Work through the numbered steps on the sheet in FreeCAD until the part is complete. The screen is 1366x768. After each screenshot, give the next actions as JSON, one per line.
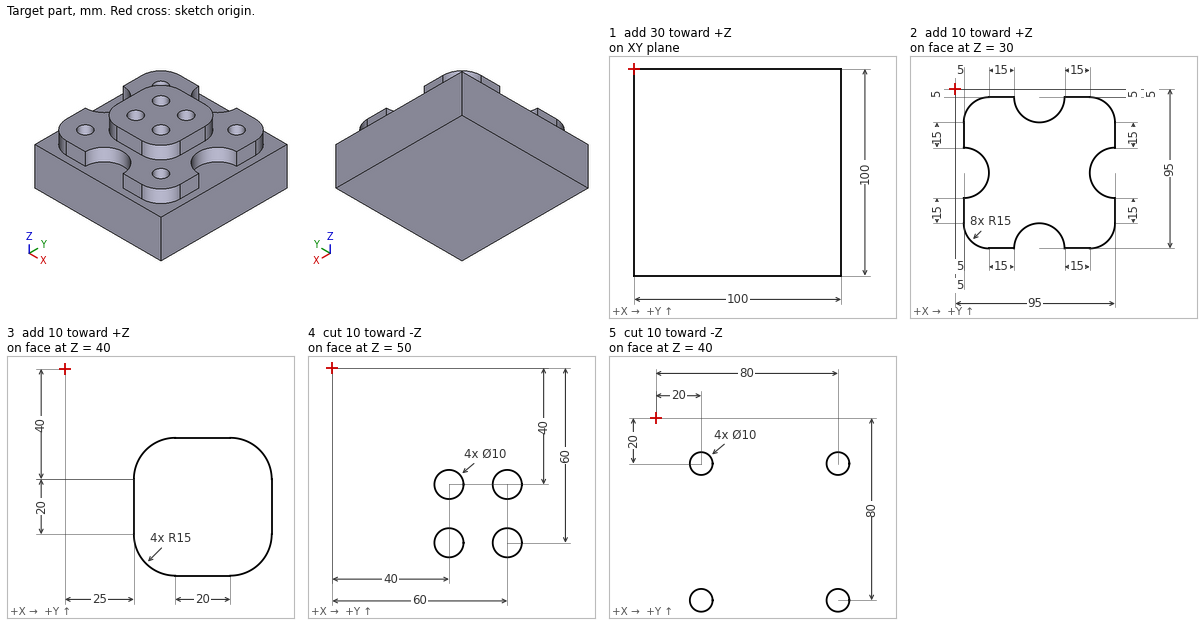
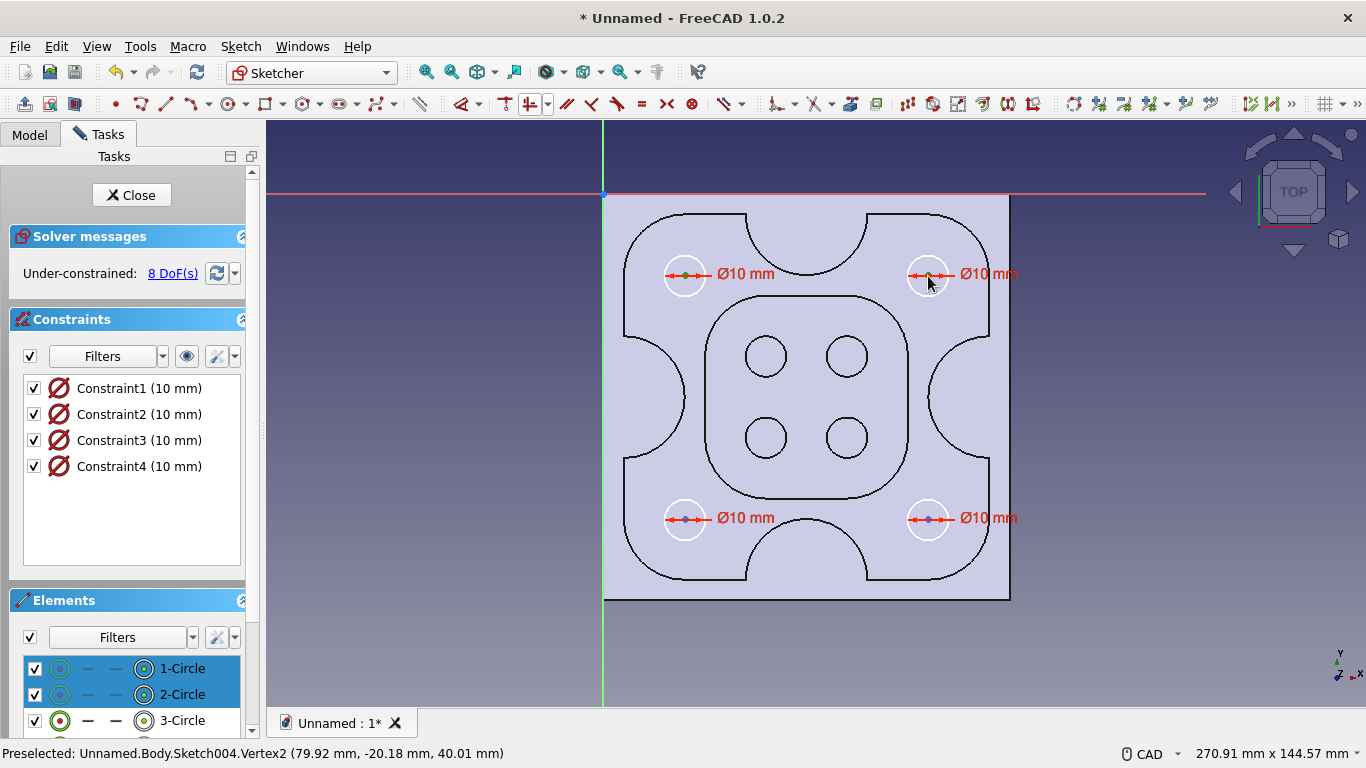
{"action": "left_click", "coordinate": [548, 104]}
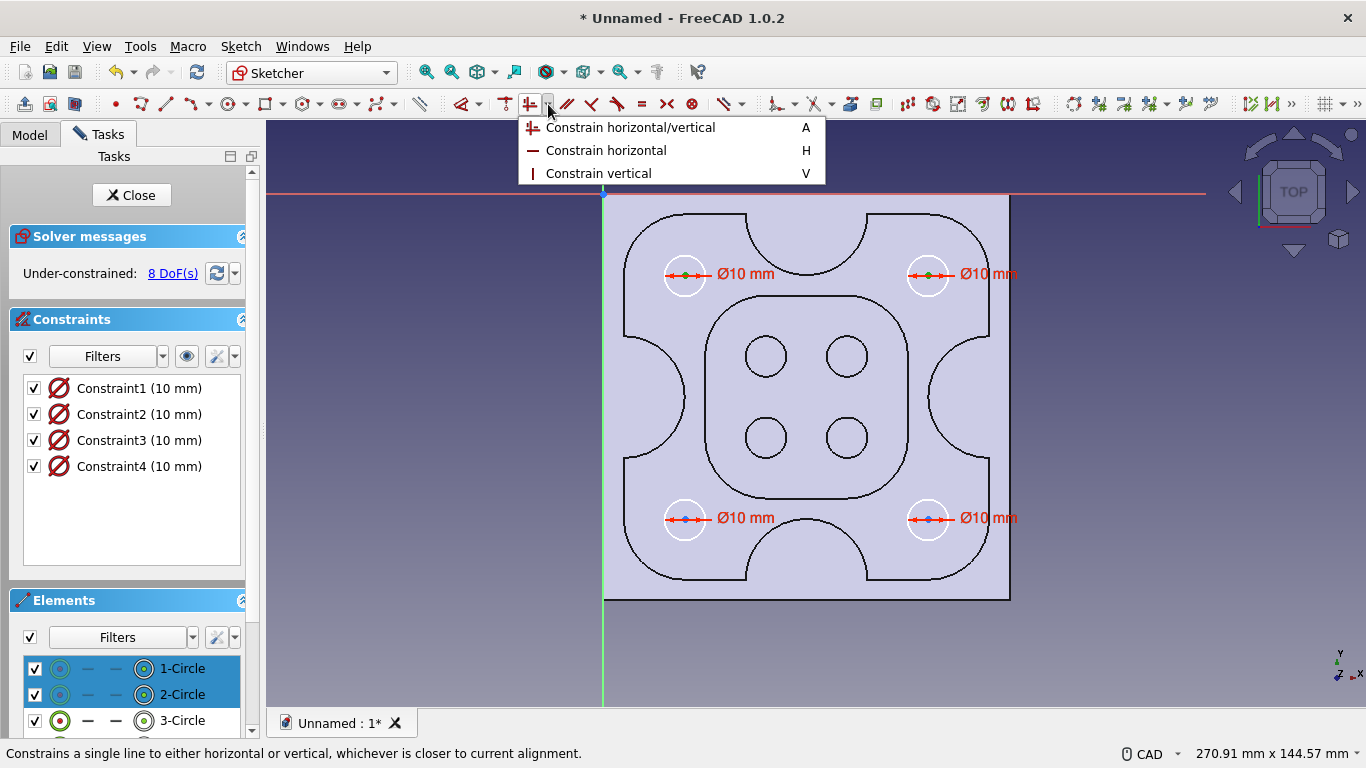
{"action": "left_click", "coordinate": [672, 150]}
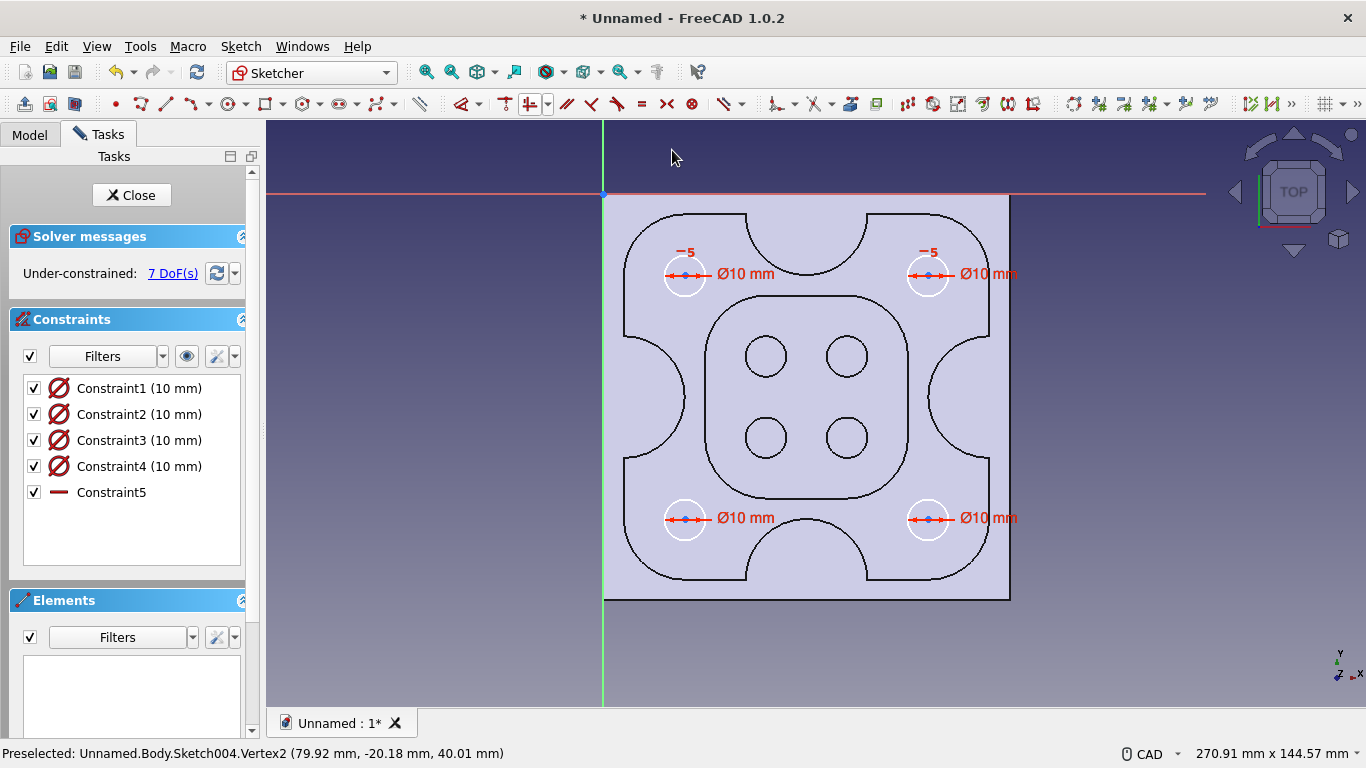
{"action": "left_click", "coordinate": [928, 276]}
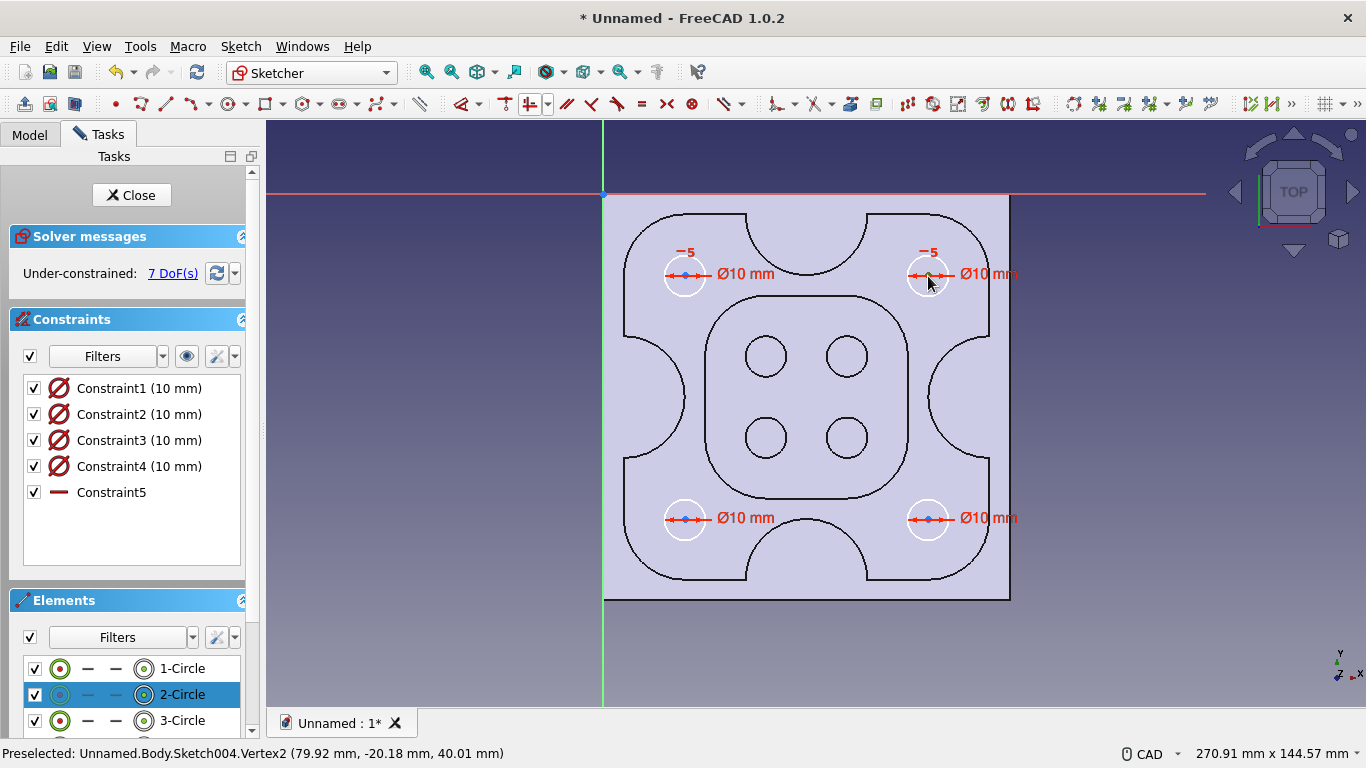
{"action": "left_click", "coordinate": [928, 520]}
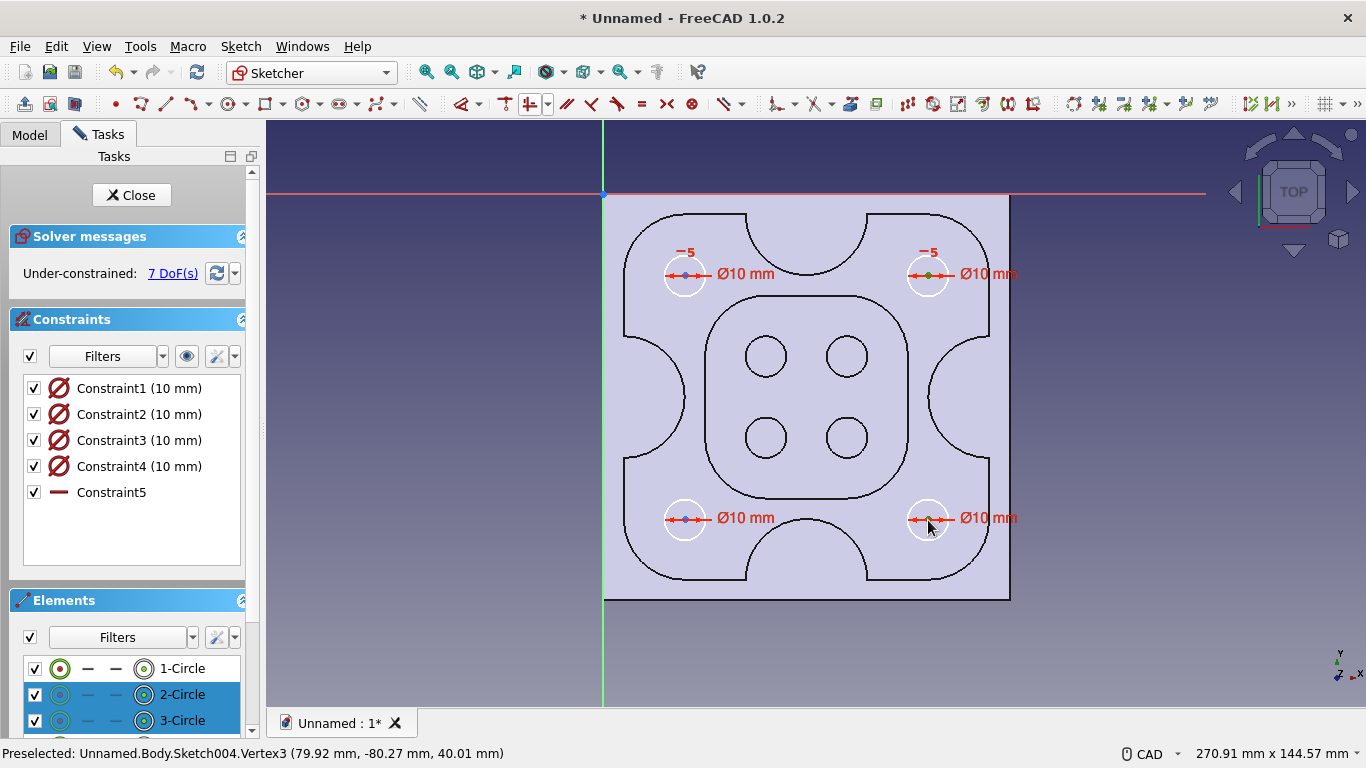
{"action": "key", "text": "v"}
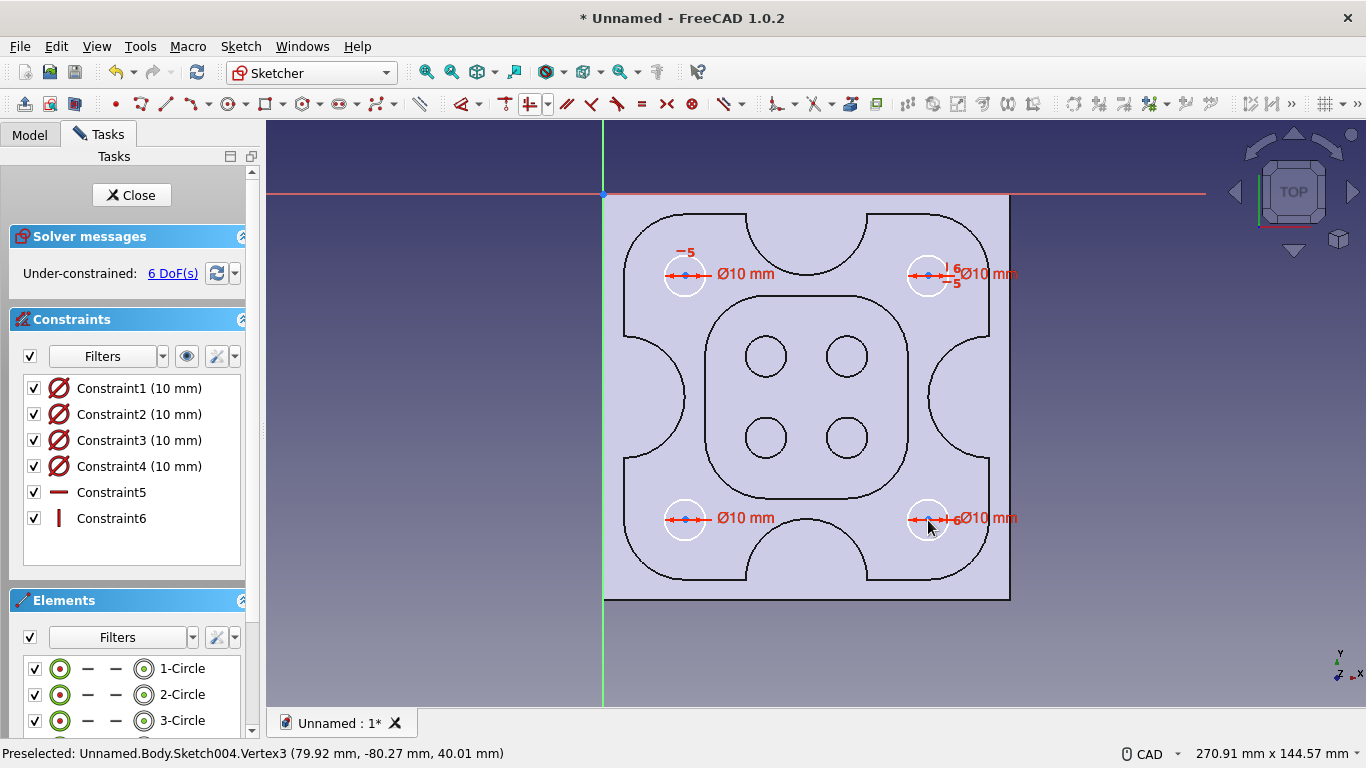
{"action": "left_click", "coordinate": [685, 276]}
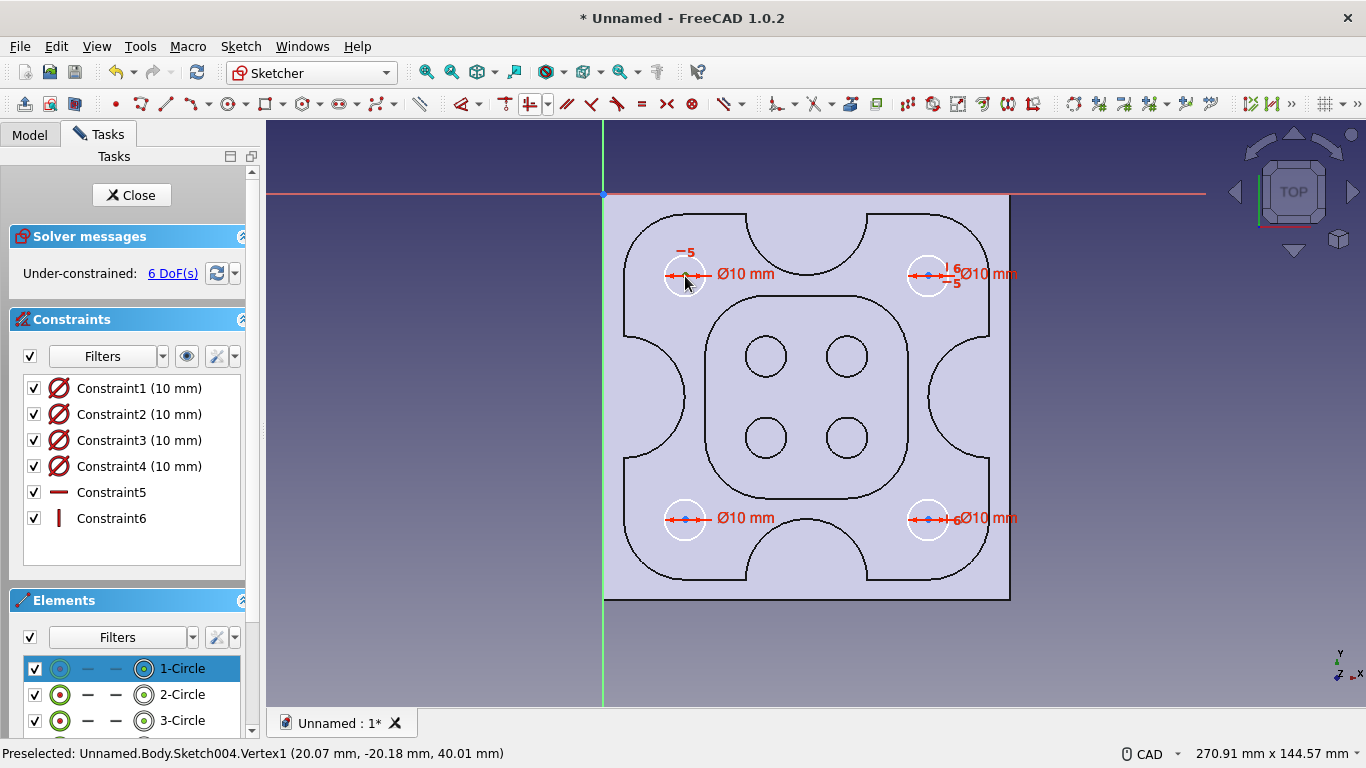
{"action": "left_click", "coordinate": [685, 520]}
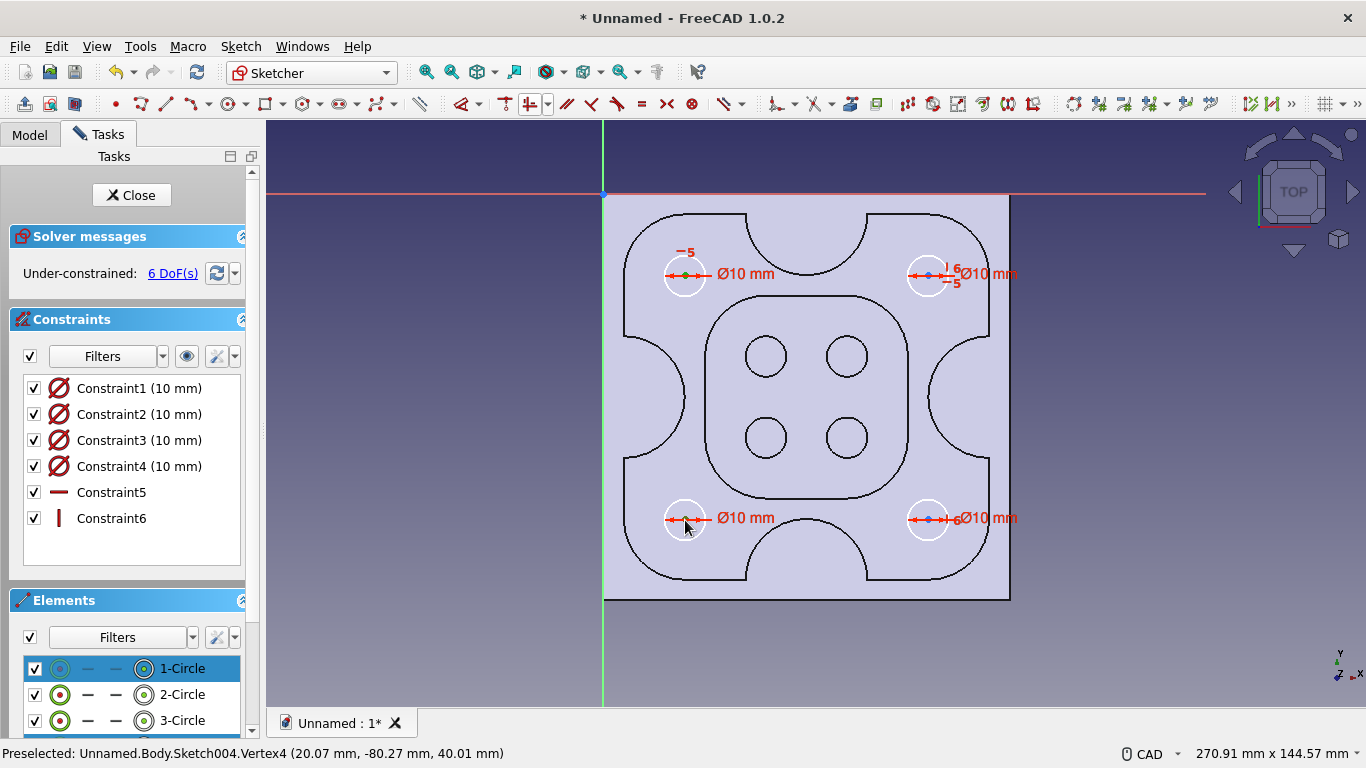
{"action": "key", "text": "v"}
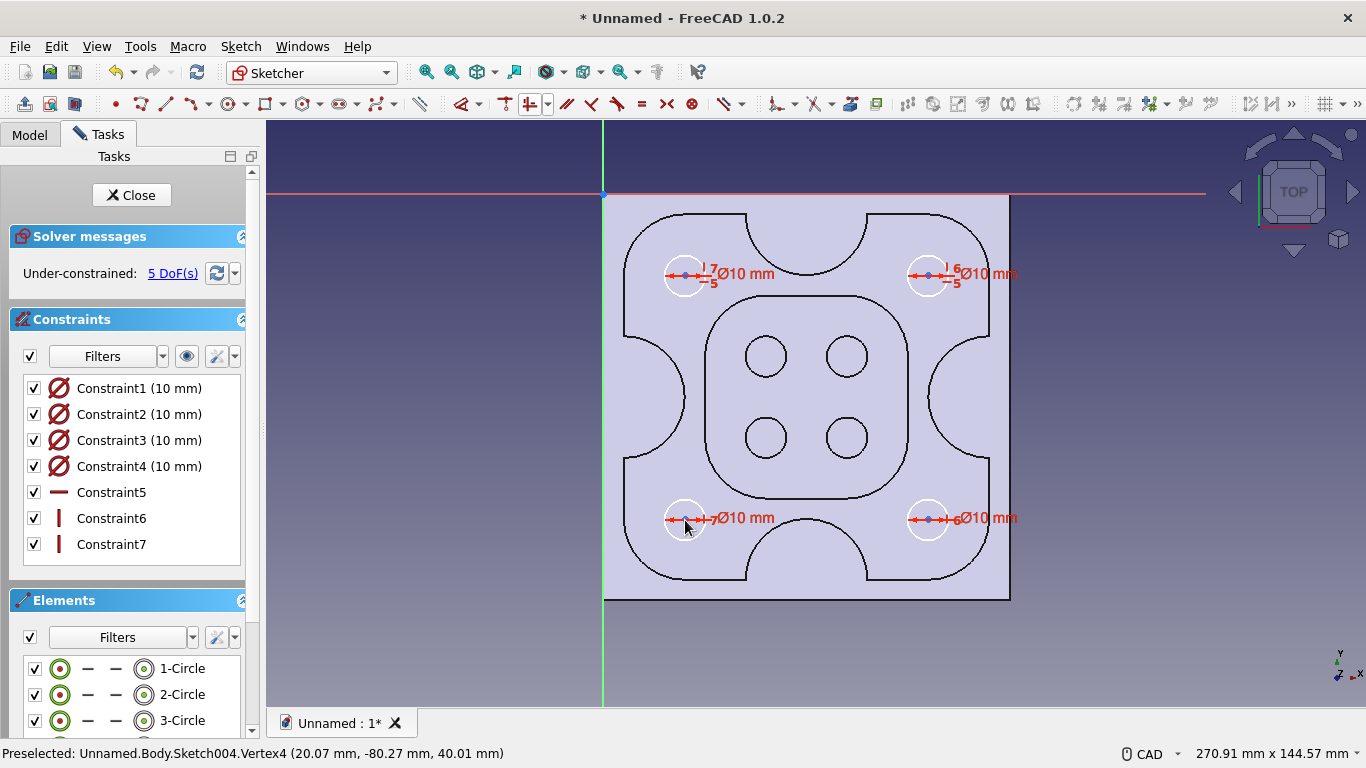
{"action": "left_click", "coordinate": [928, 520]}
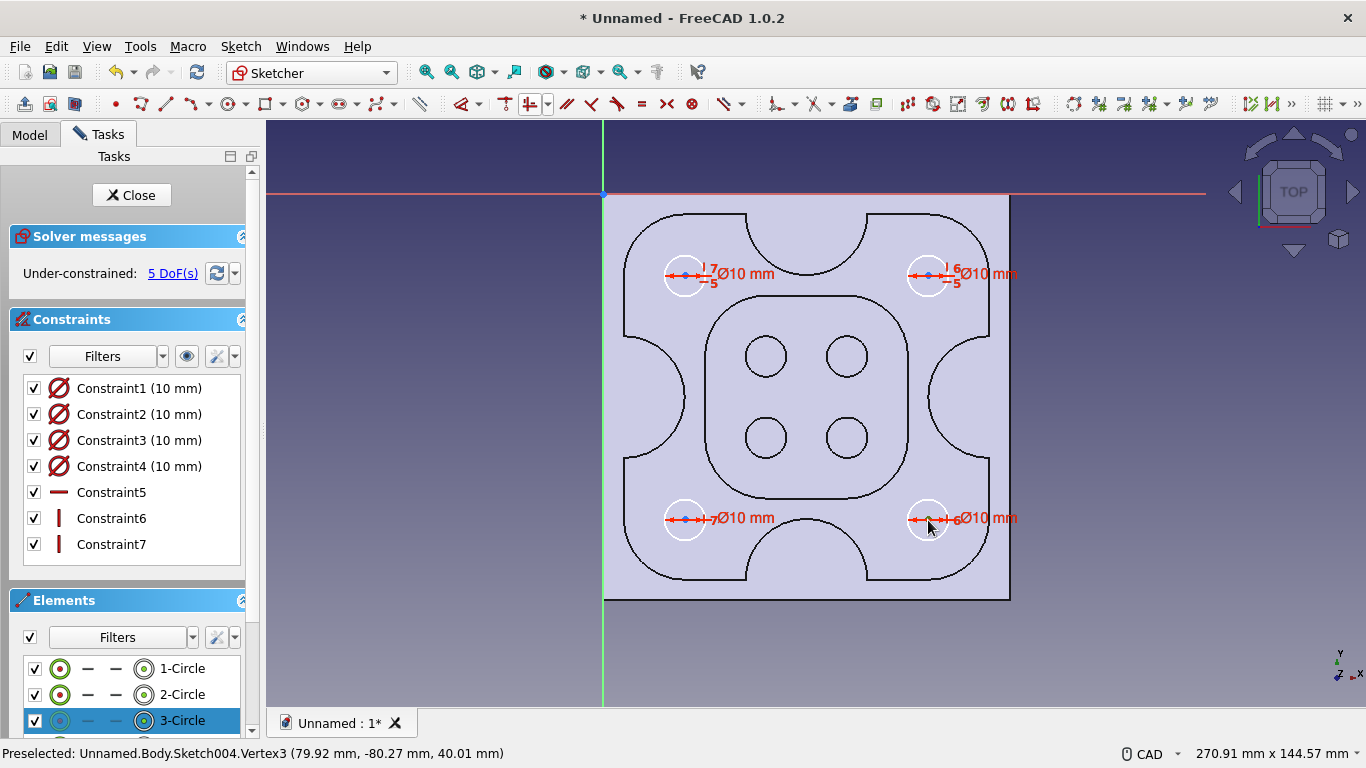
{"action": "left_click", "coordinate": [685, 520]}